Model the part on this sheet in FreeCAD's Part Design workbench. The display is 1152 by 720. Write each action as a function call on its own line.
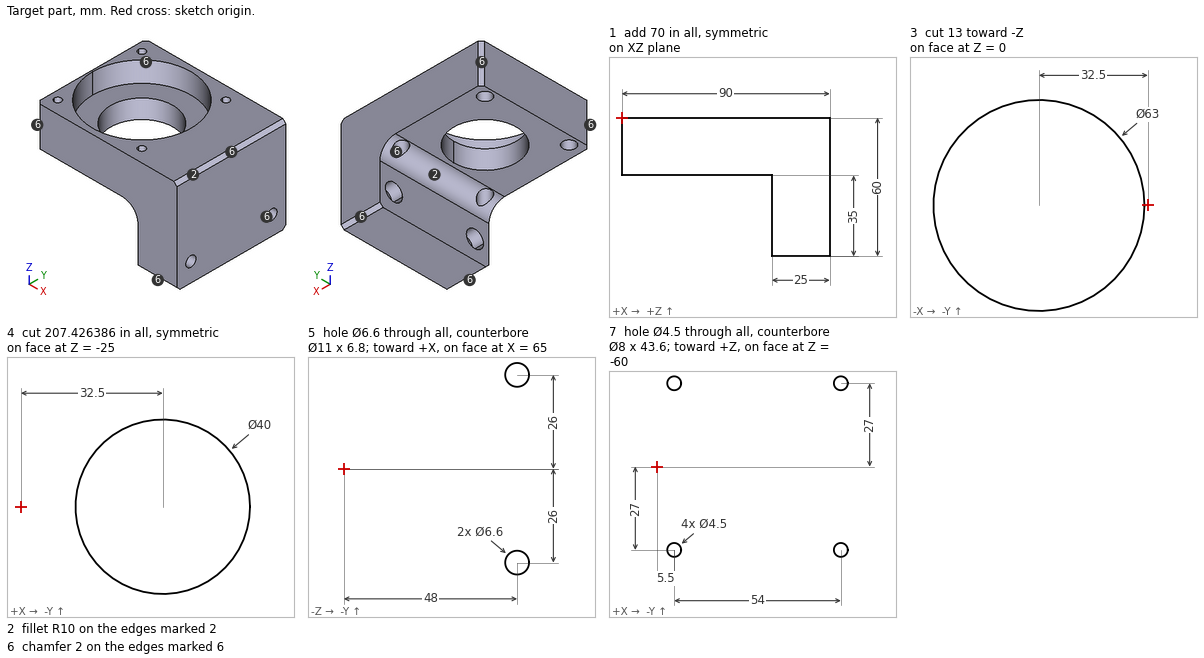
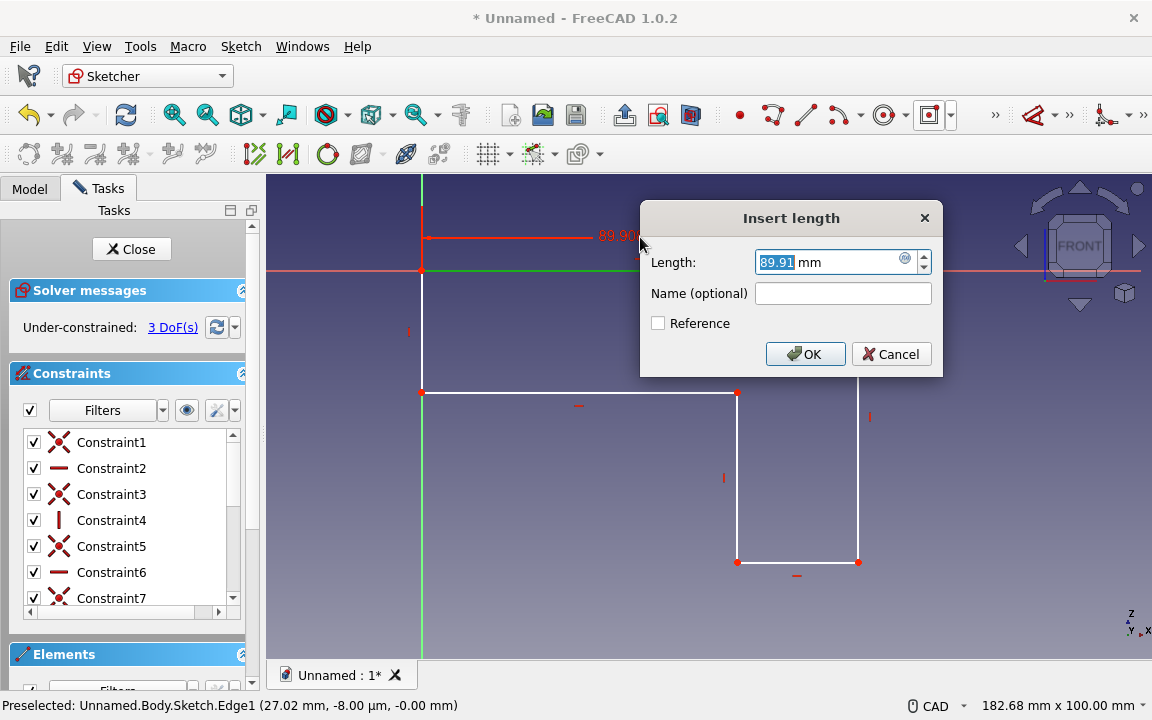
text(90)
key(Return)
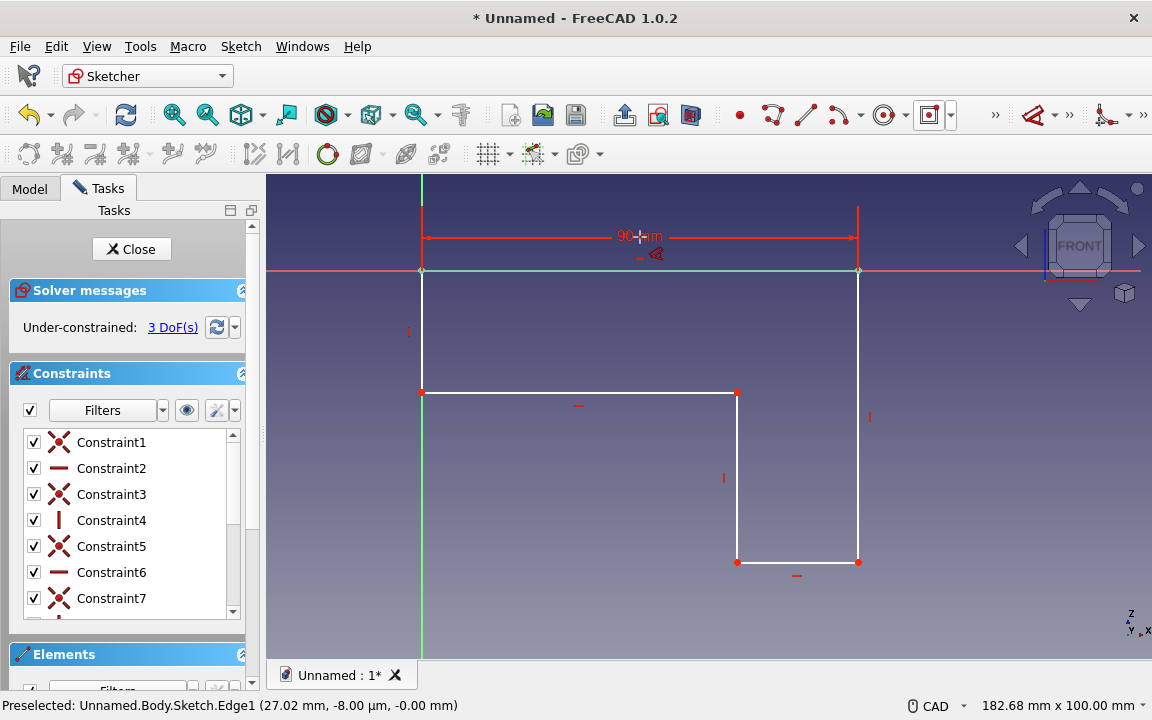
click(858, 358)
click(892, 417)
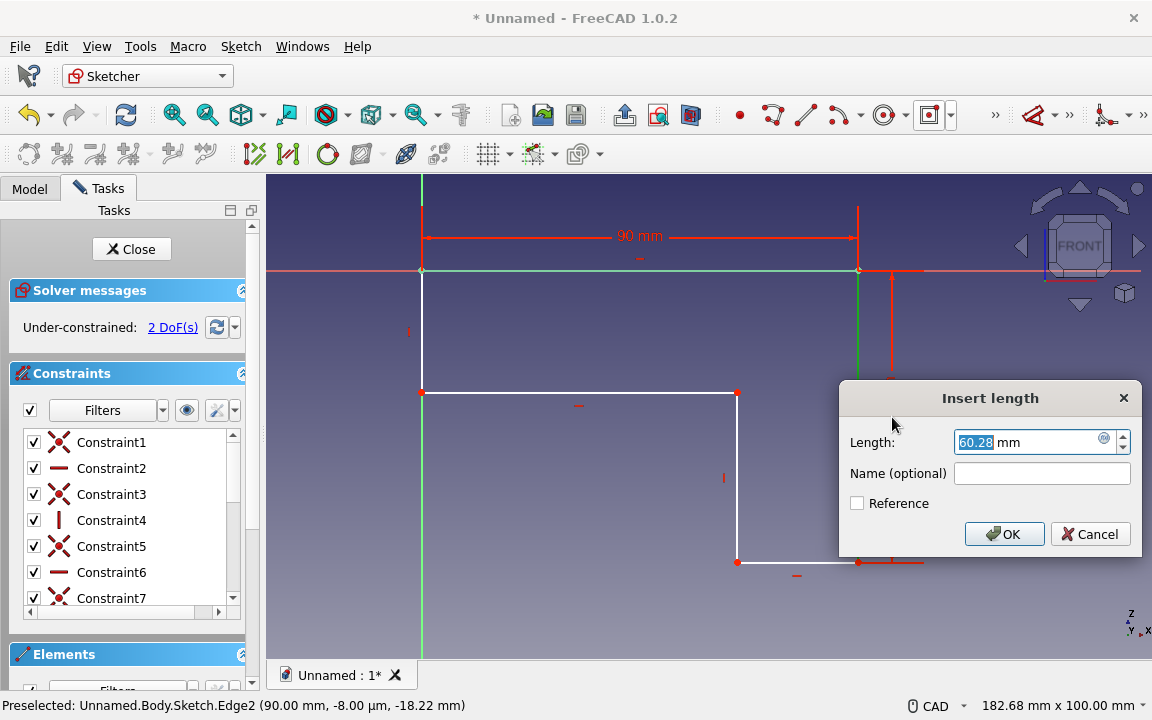
text(60)
key(Return)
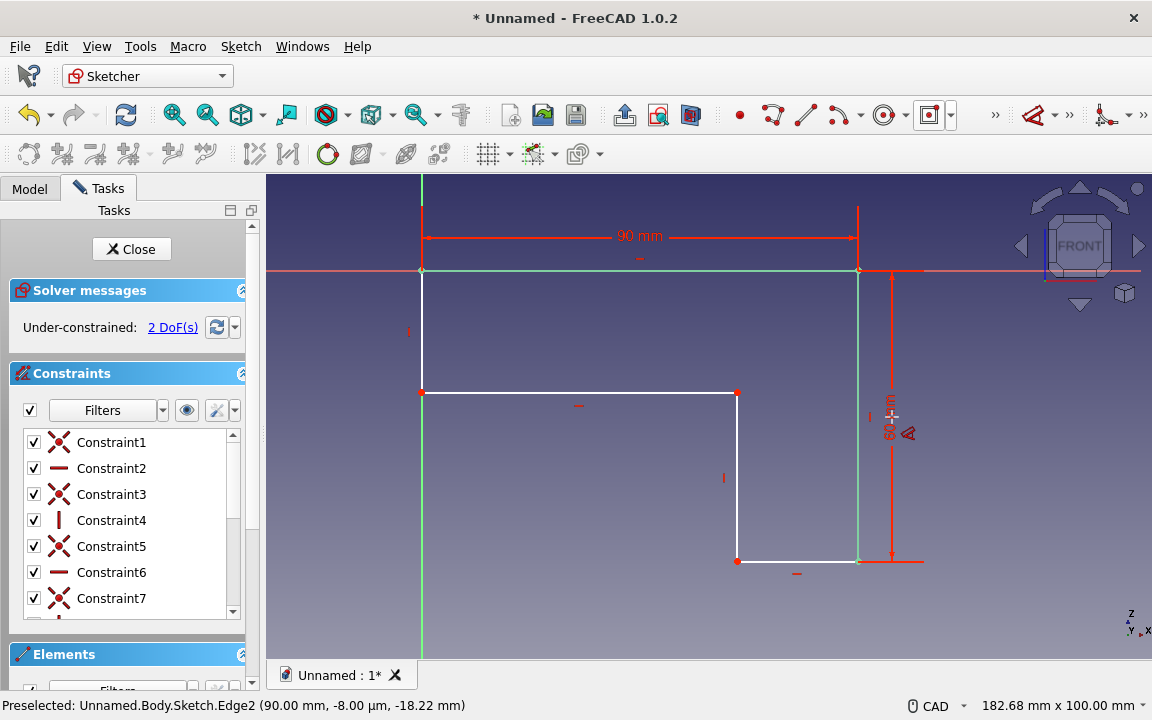
click(822, 562)
click(798, 596)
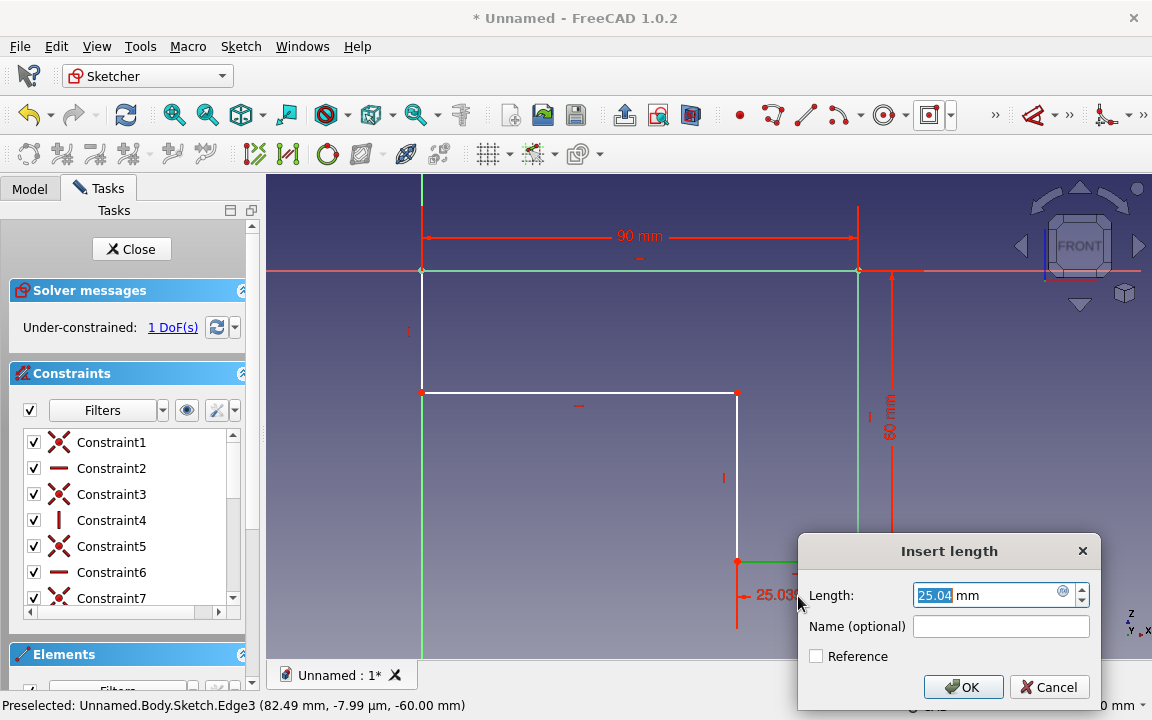
text(25)
key(Return)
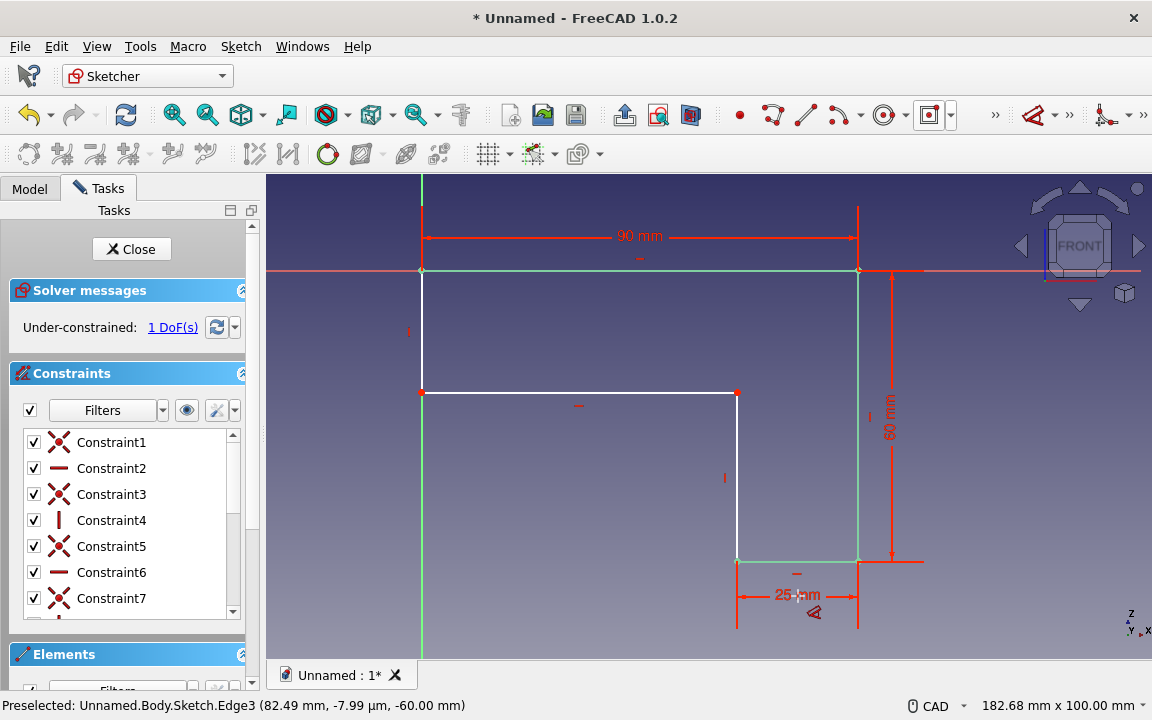
click(737, 511)
click(771, 477)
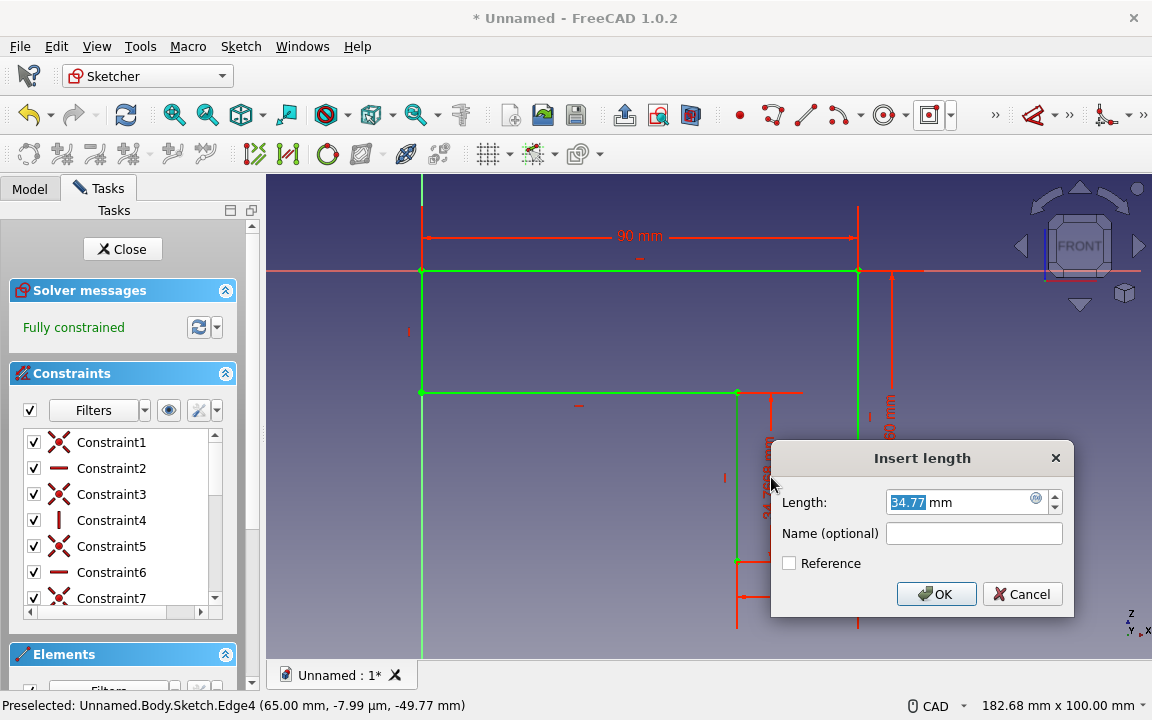
text(35)
key(Return)
key(Escape)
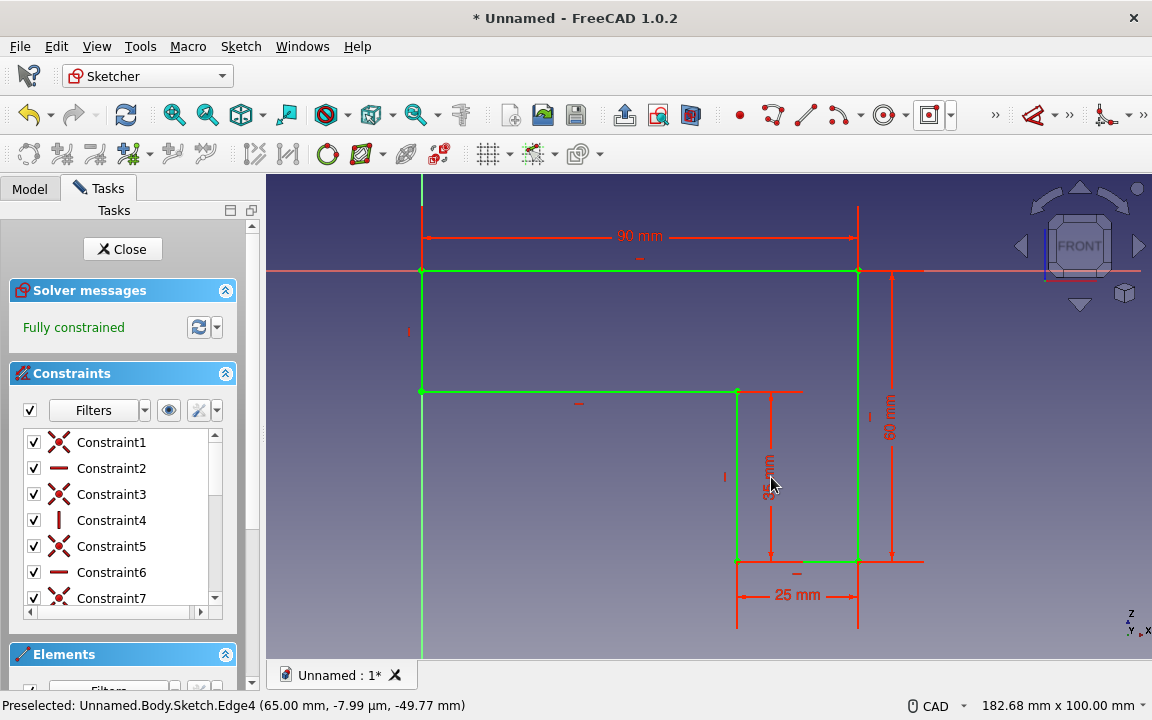
click(123, 249)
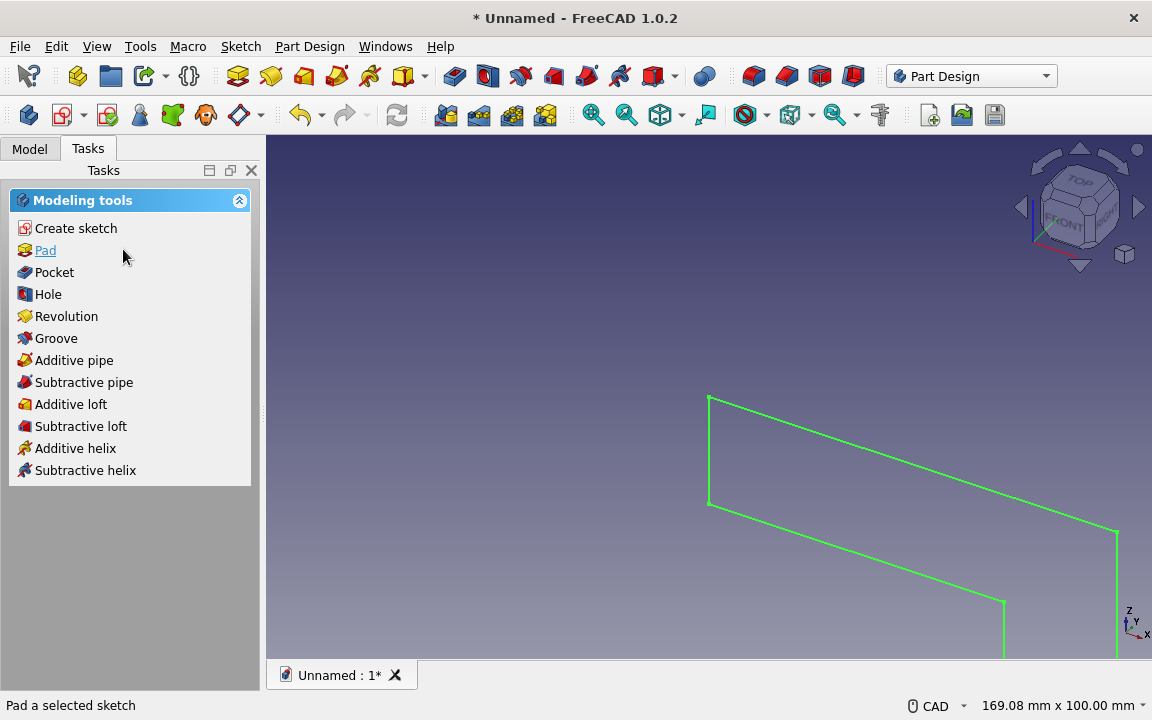
click(238, 76)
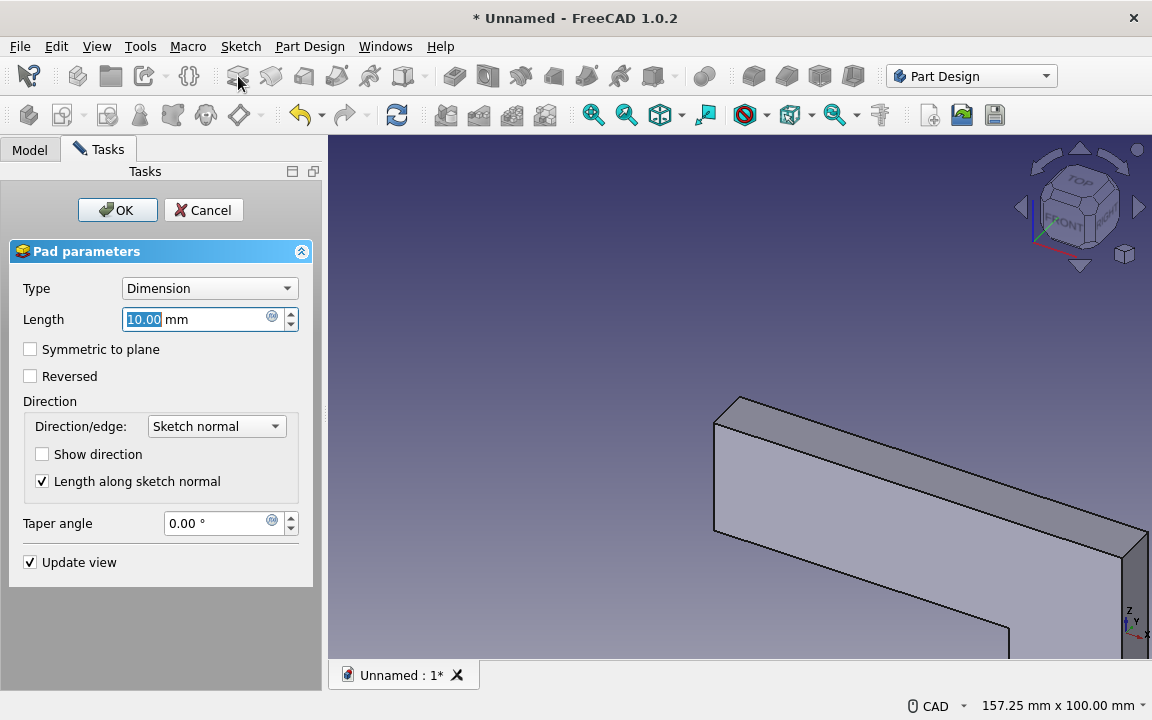
text(70)
key(Tab)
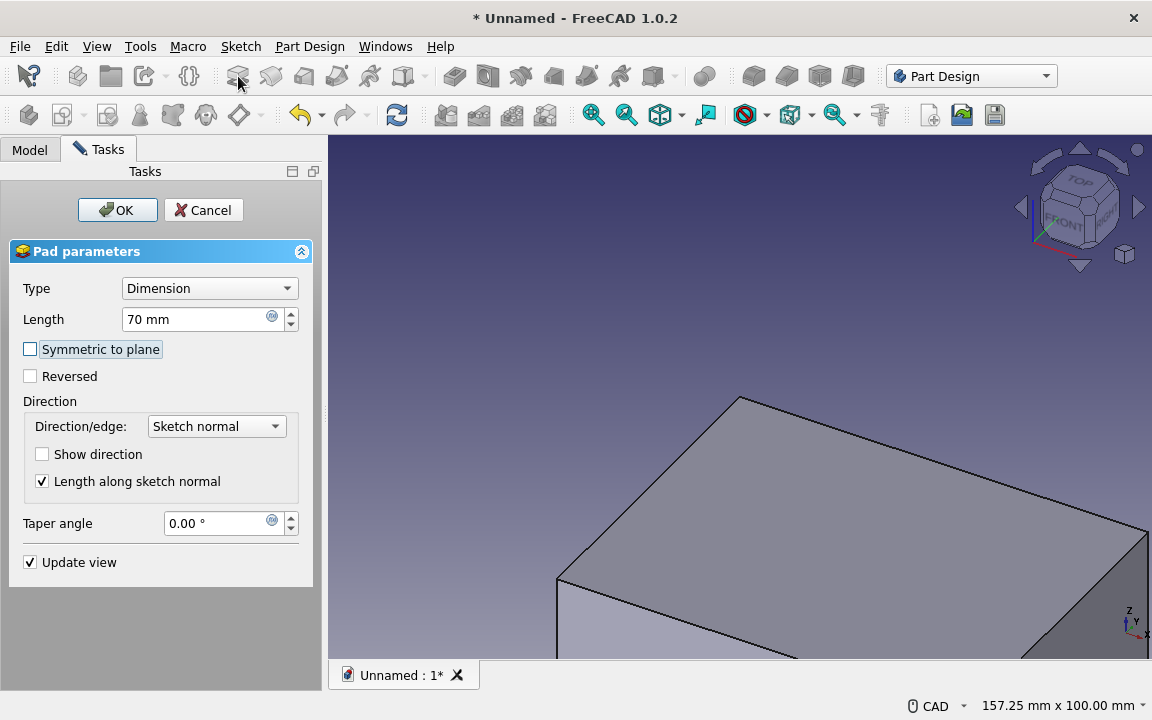
click(31, 349)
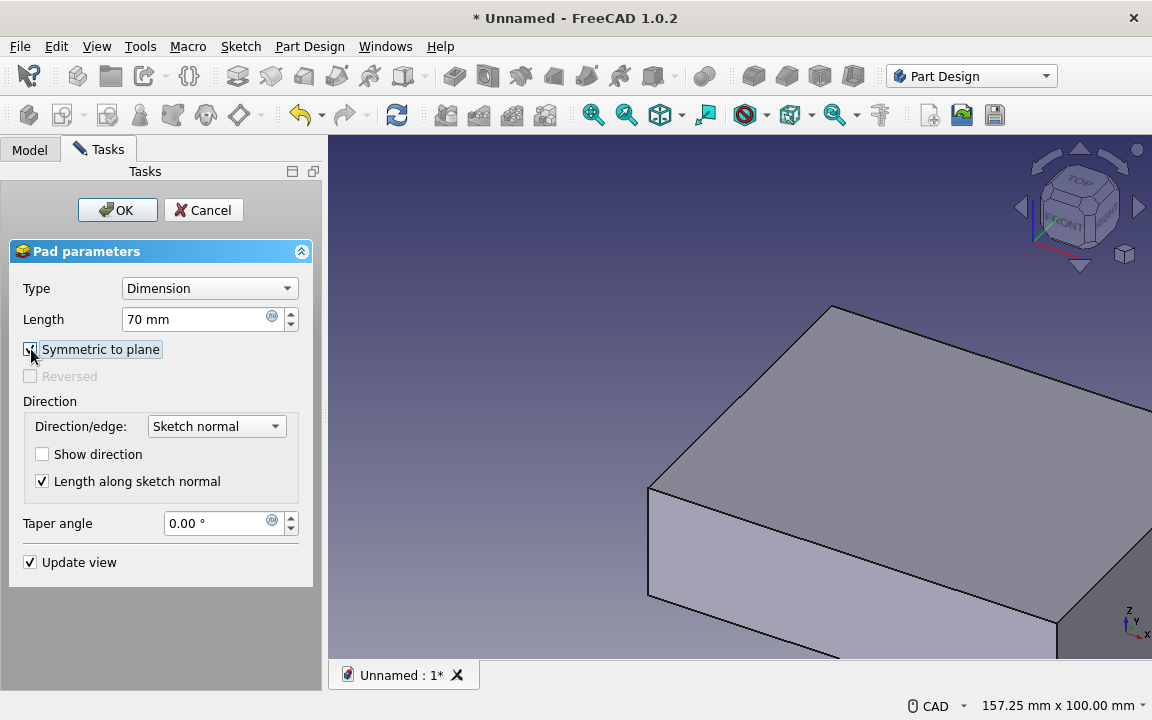
click(118, 210)